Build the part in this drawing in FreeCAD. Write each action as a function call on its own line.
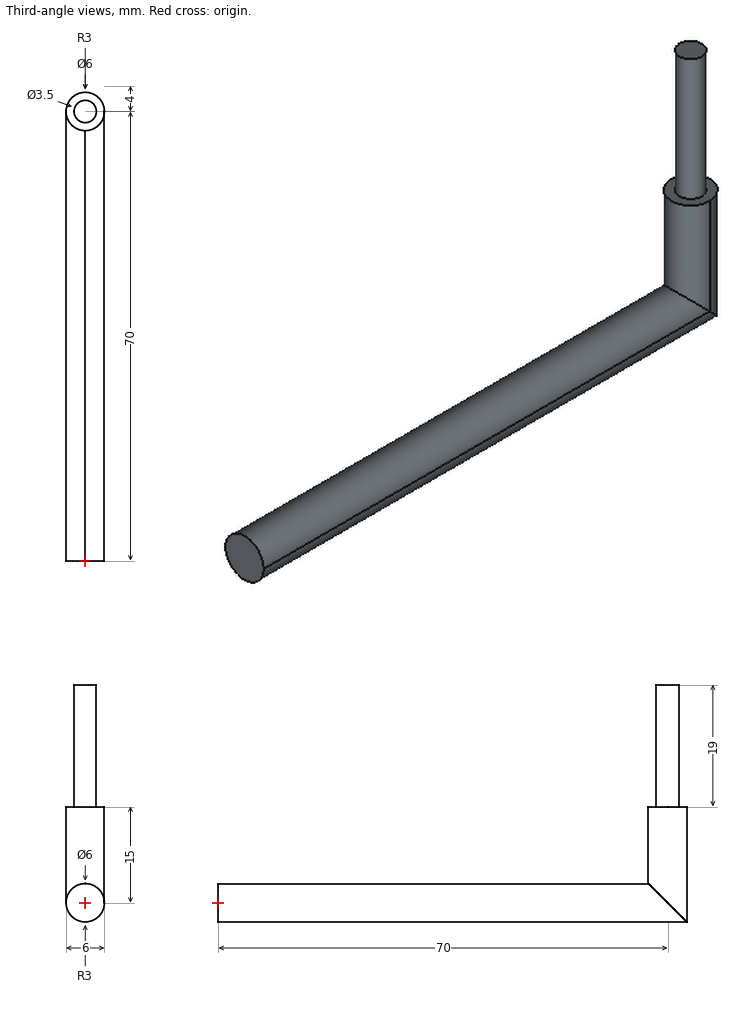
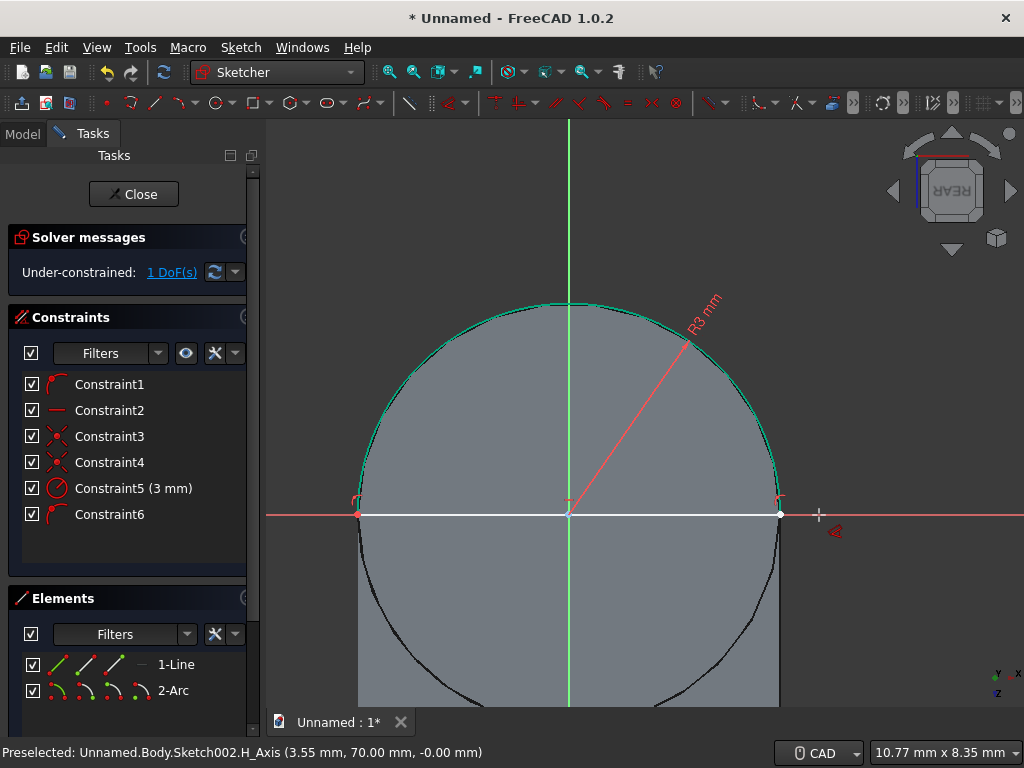
click(485, 515)
click(472, 549)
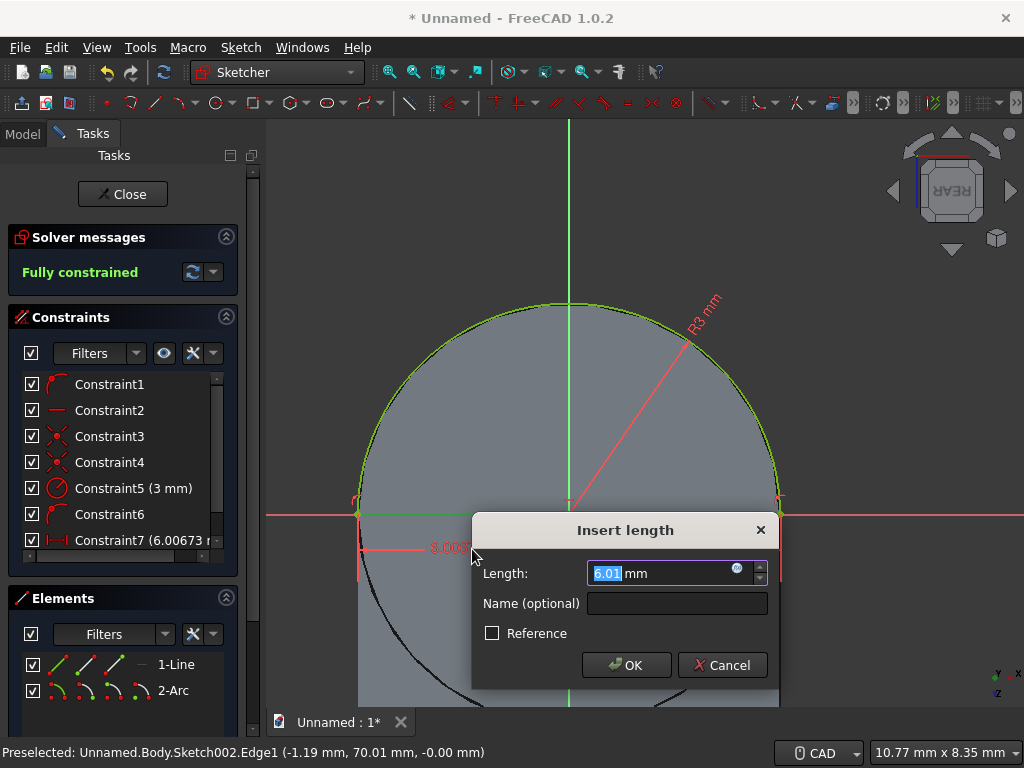
text(6)
key(Return)
key(Escape)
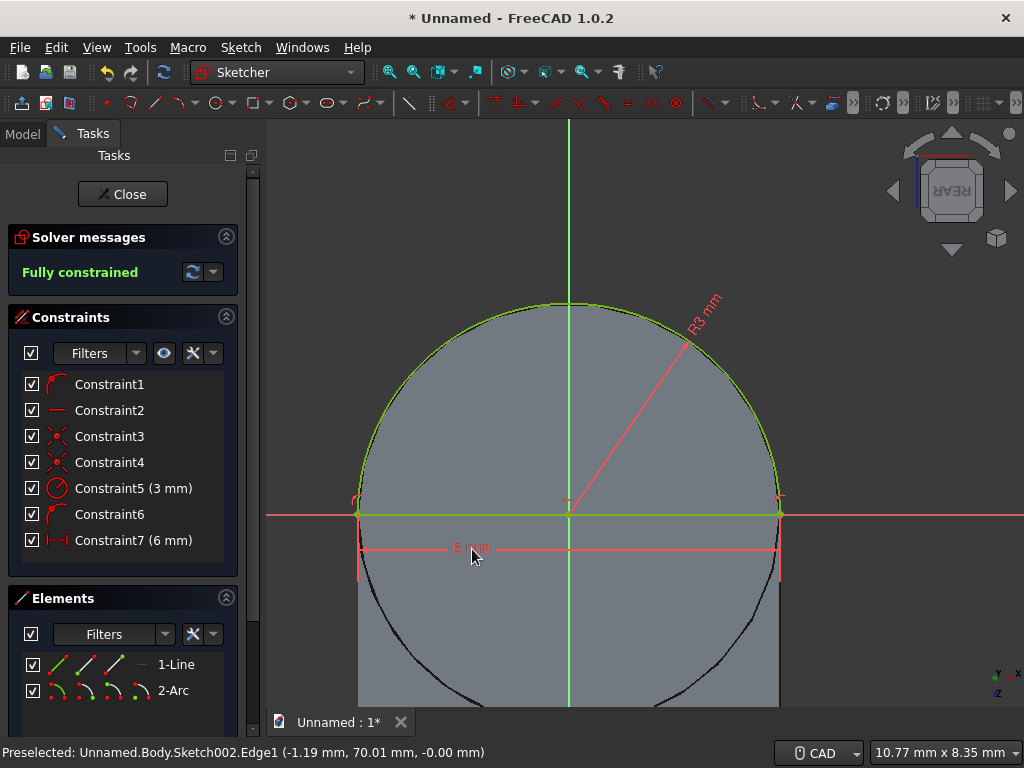
click(123, 194)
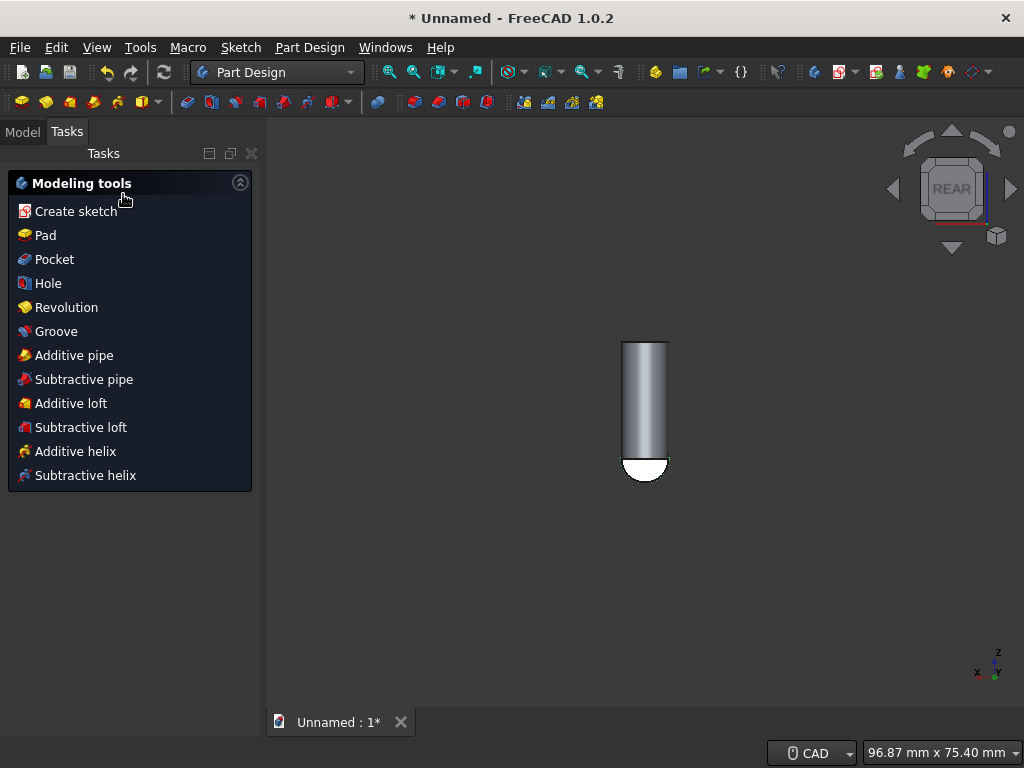
click(22, 102)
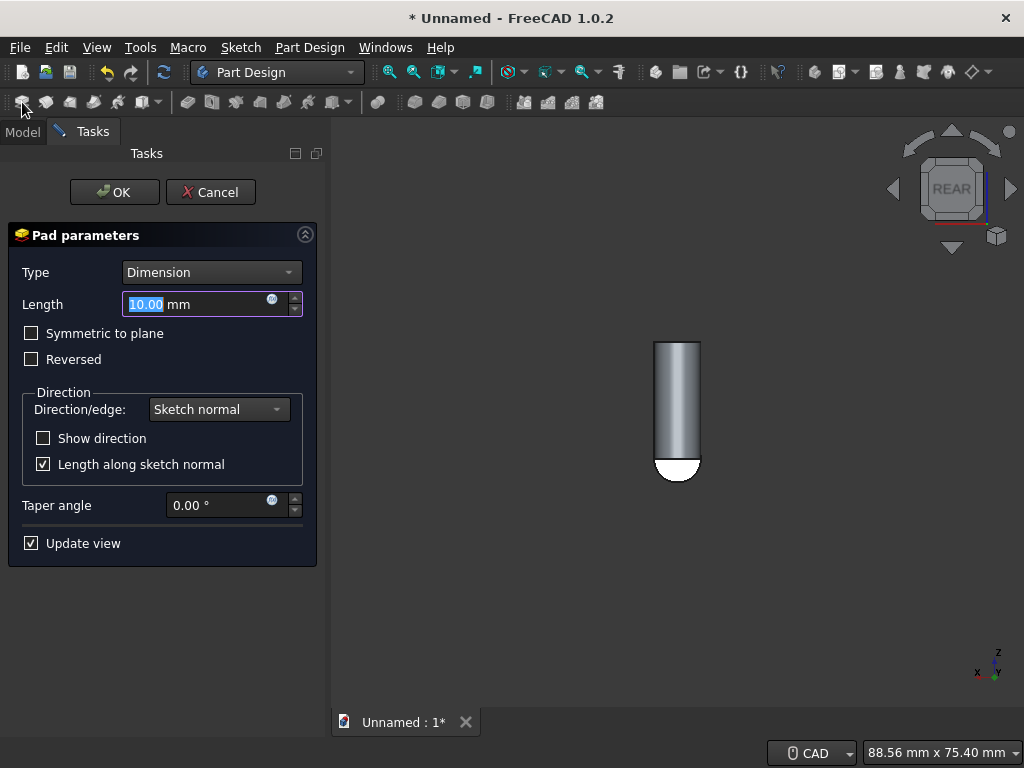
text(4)
key(Tab)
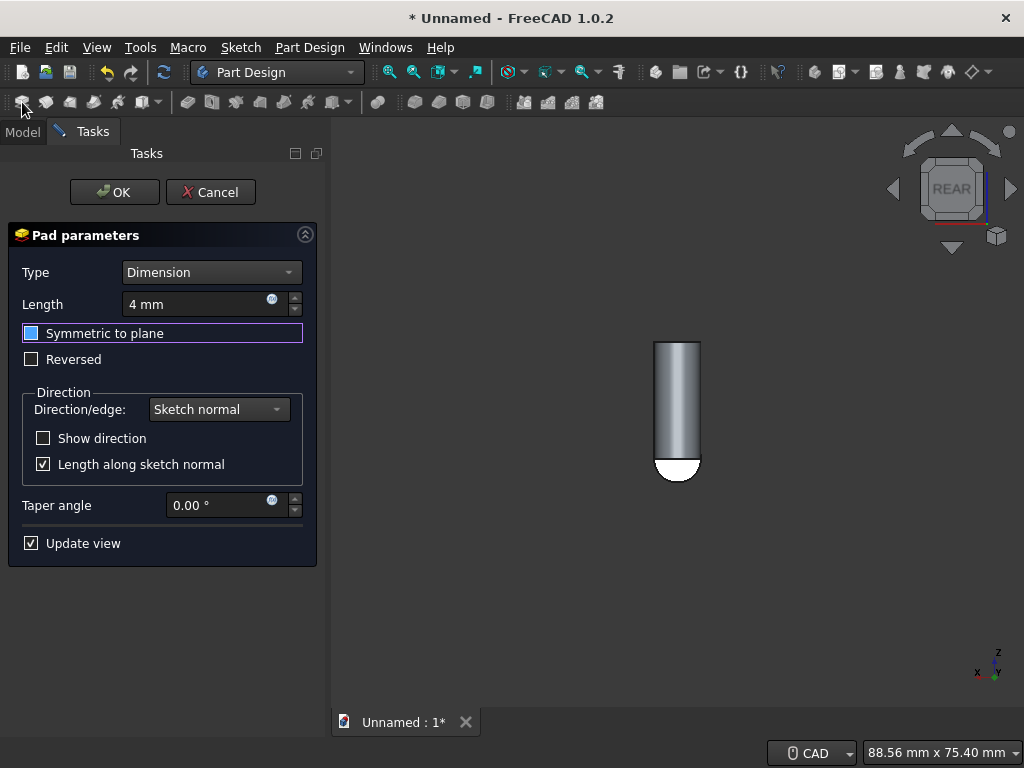
click(115, 192)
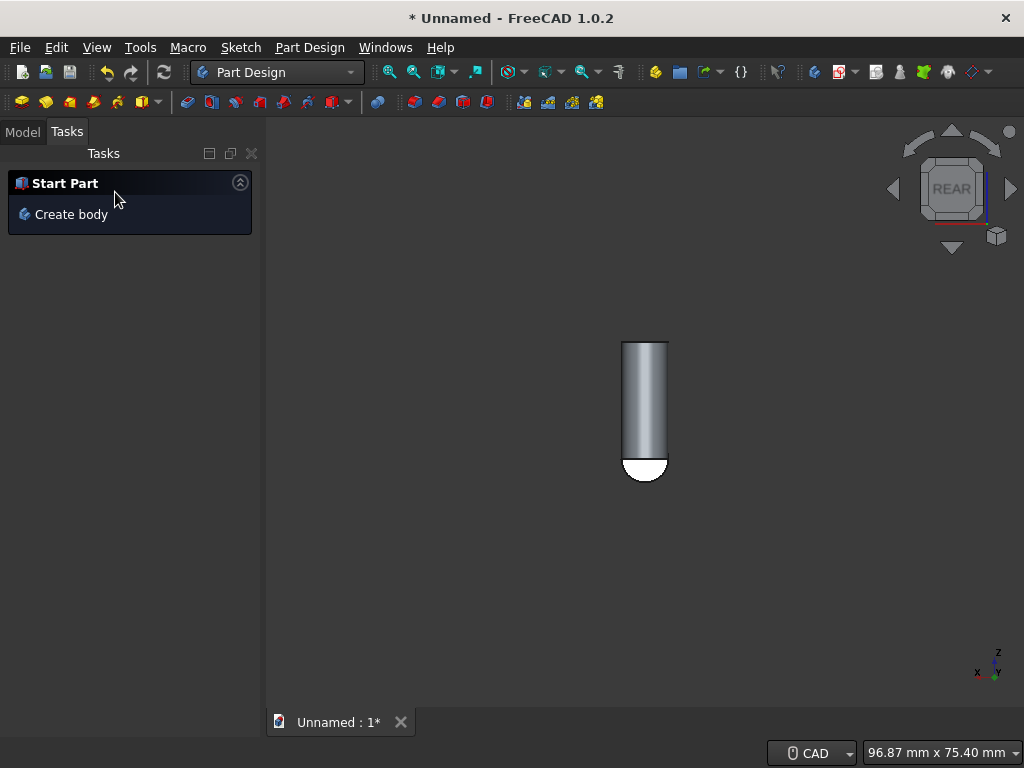
key(v)
key(f)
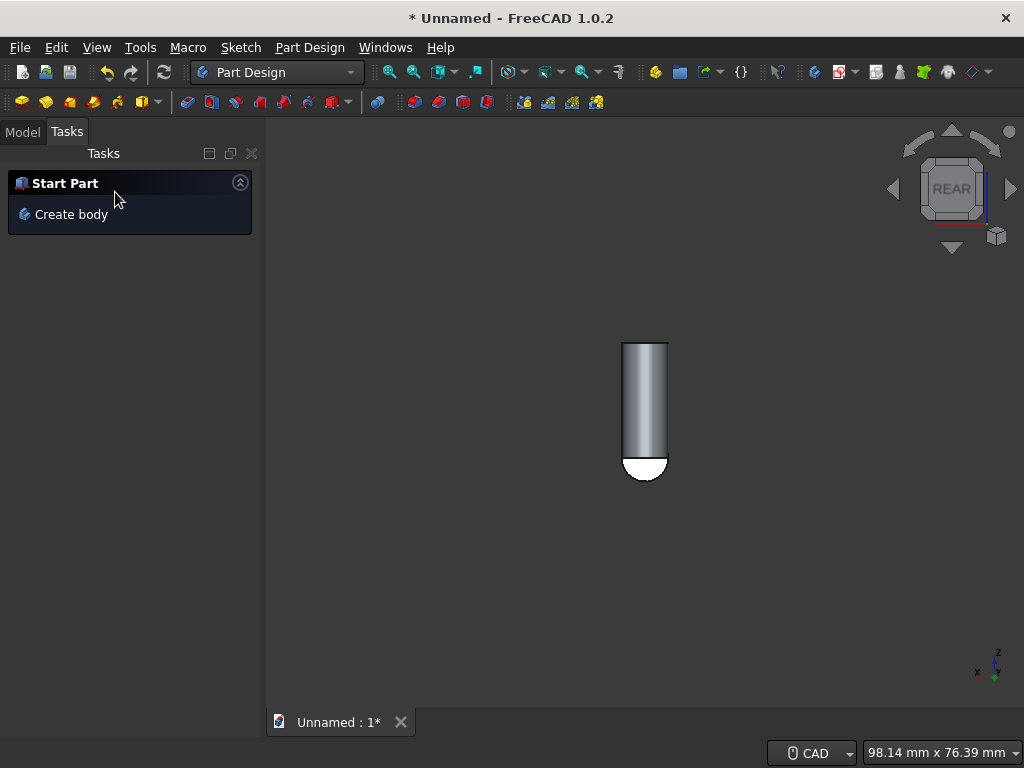
key(0)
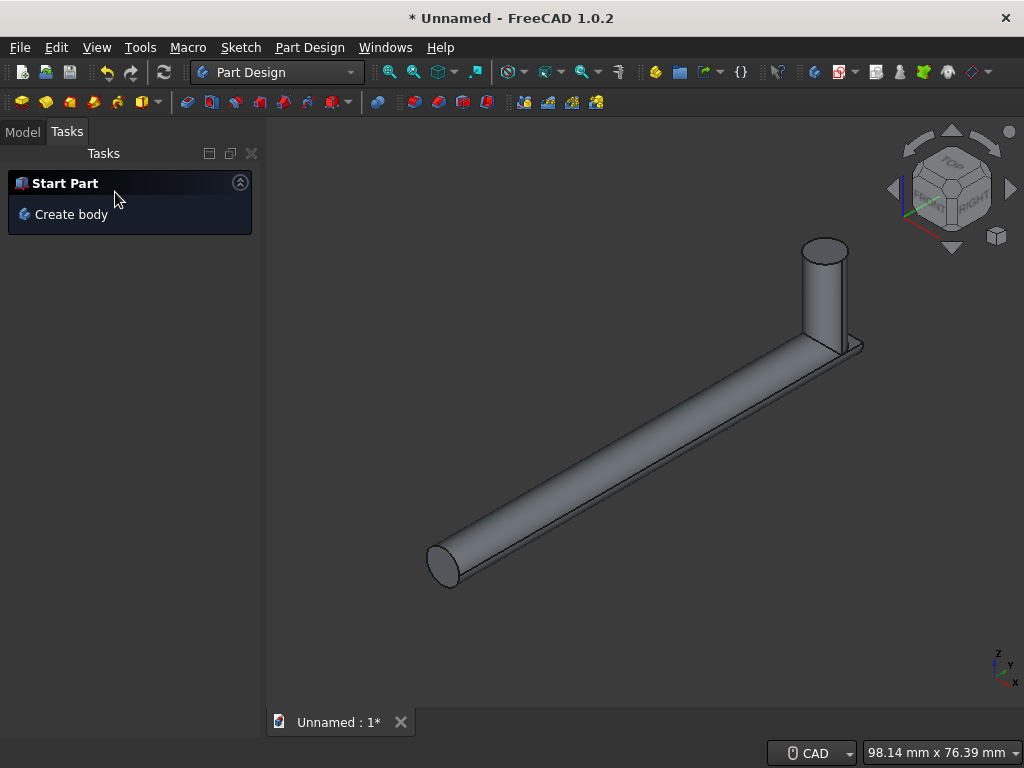
click(825, 250)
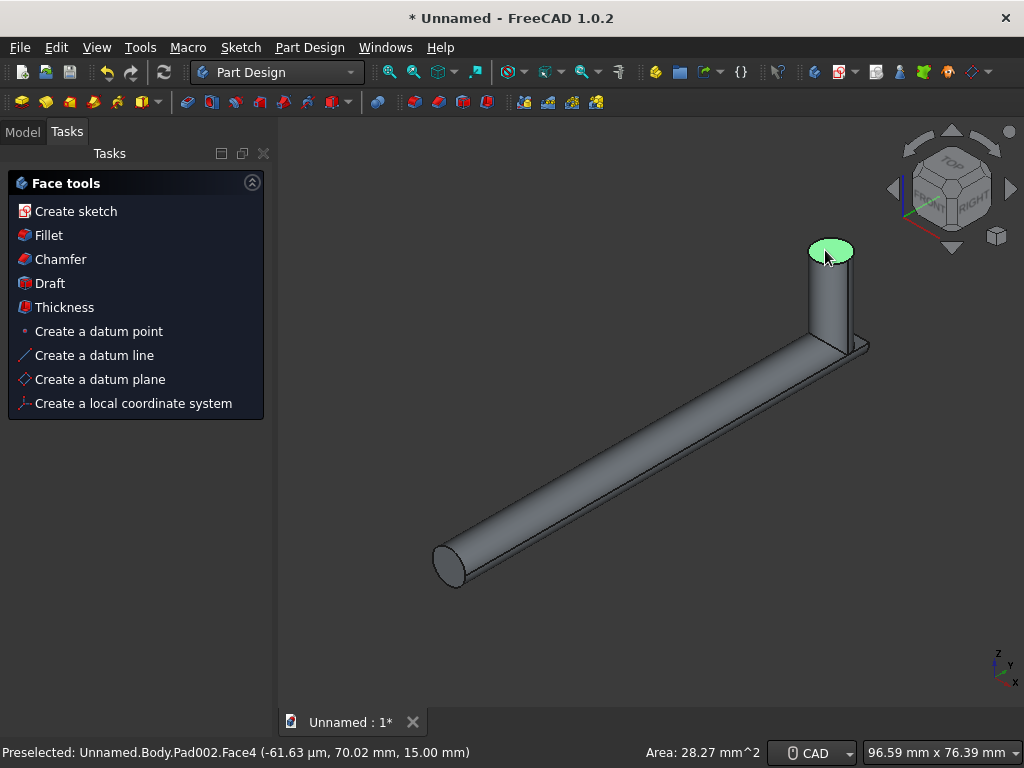
click(840, 72)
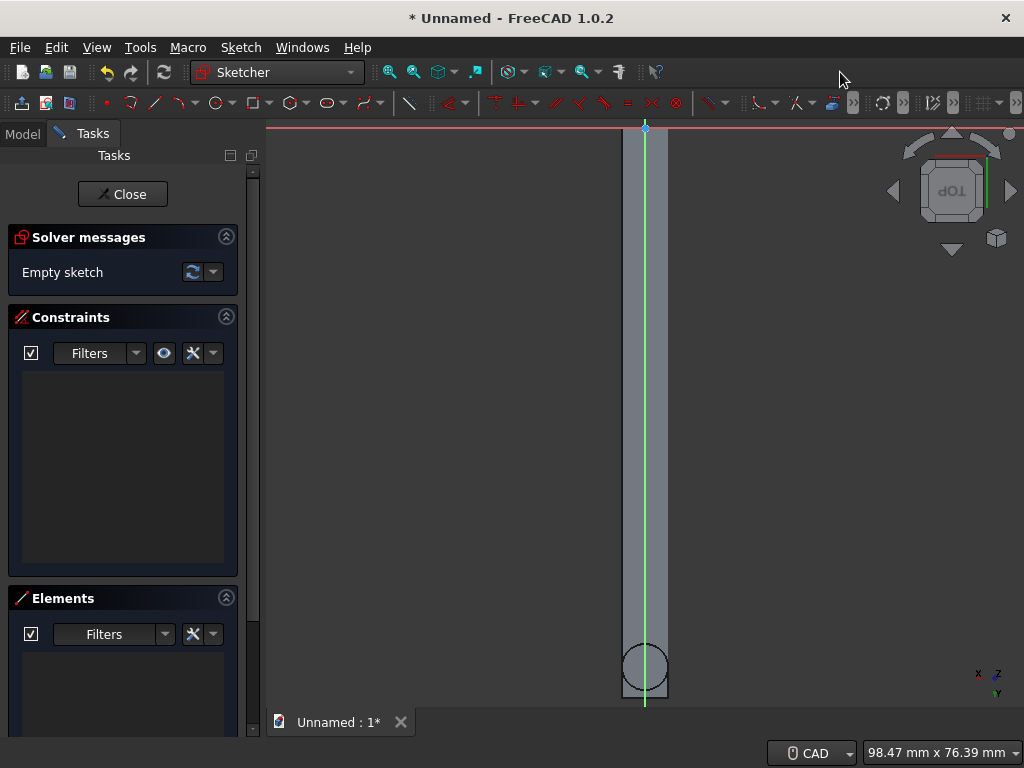
scroll(576, 413, down, 5)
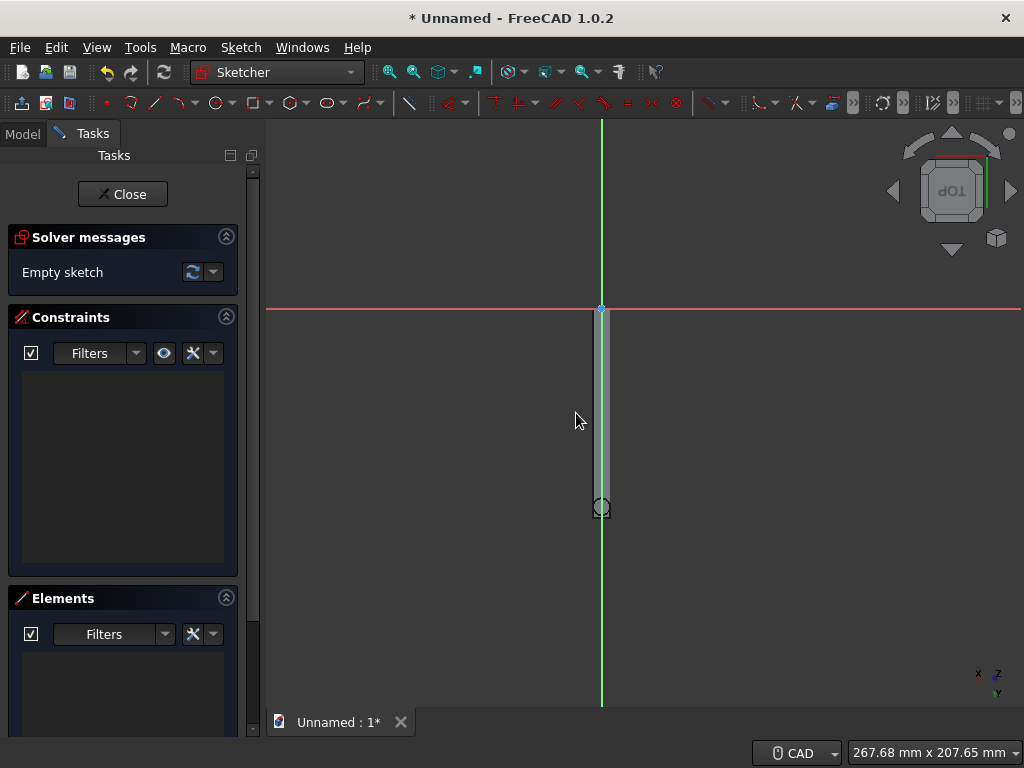
scroll(603, 518, up, 15)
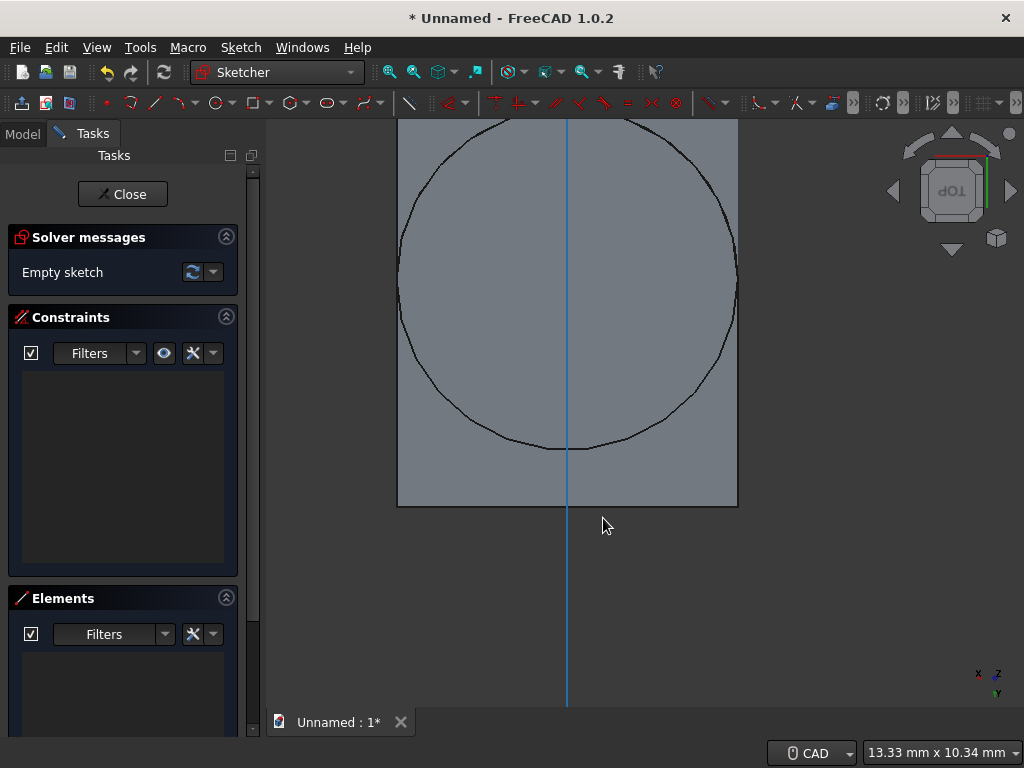
click(132, 104)